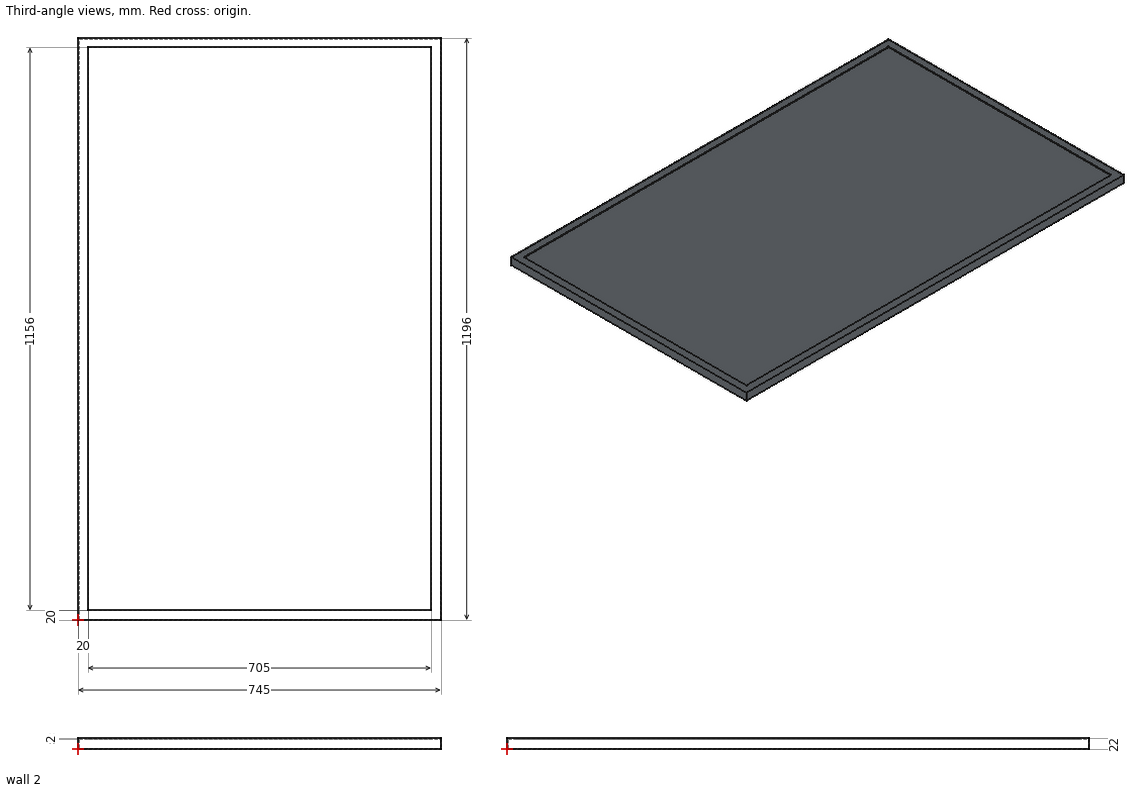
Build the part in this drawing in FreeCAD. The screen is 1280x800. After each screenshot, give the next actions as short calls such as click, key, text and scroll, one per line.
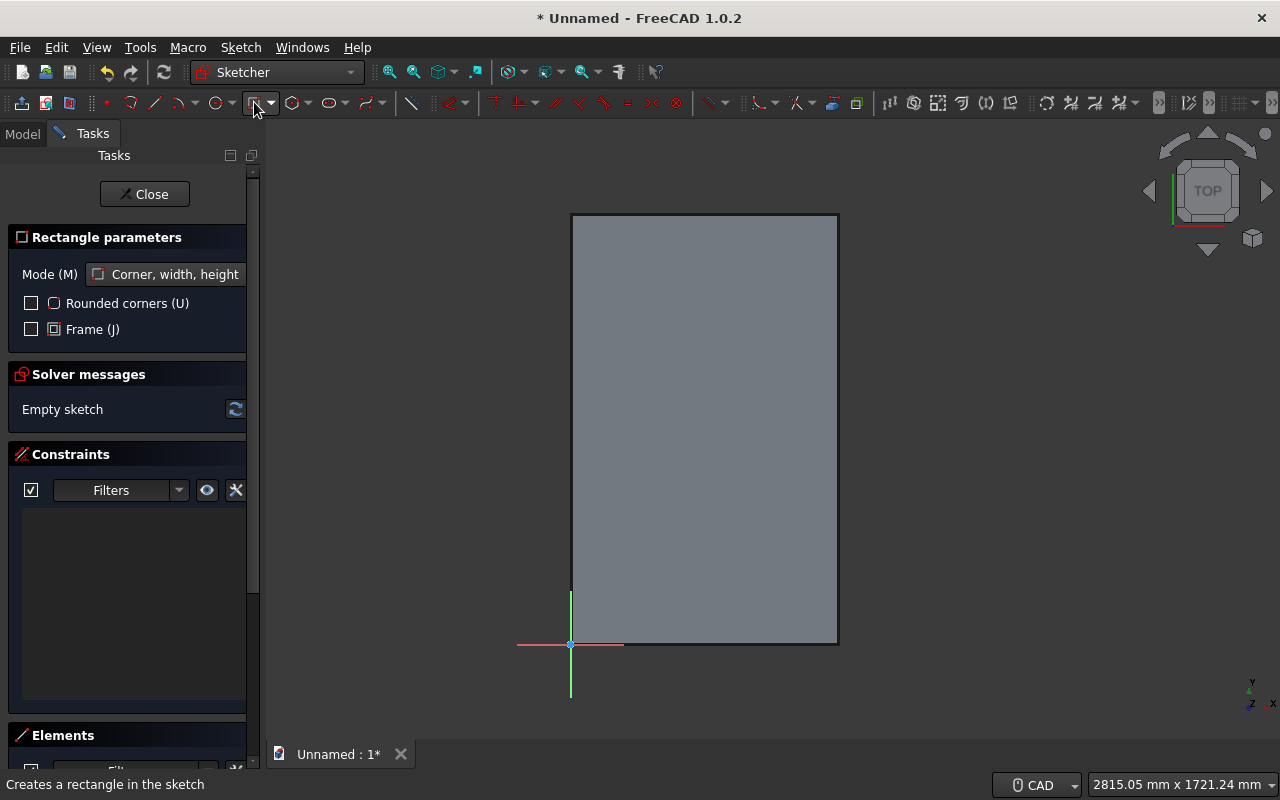
click(571, 645)
move(839, 214)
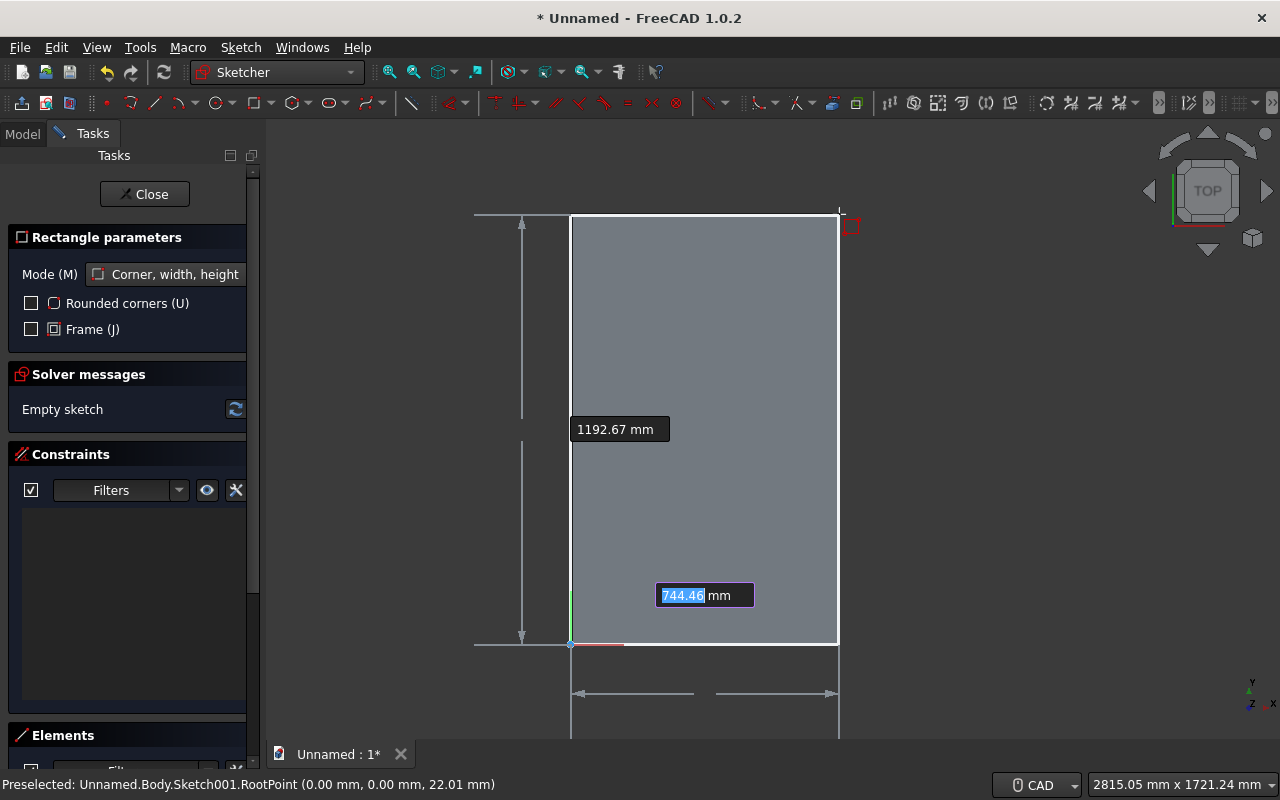
text(745)
key(Tab)
text(1196)
key(Return)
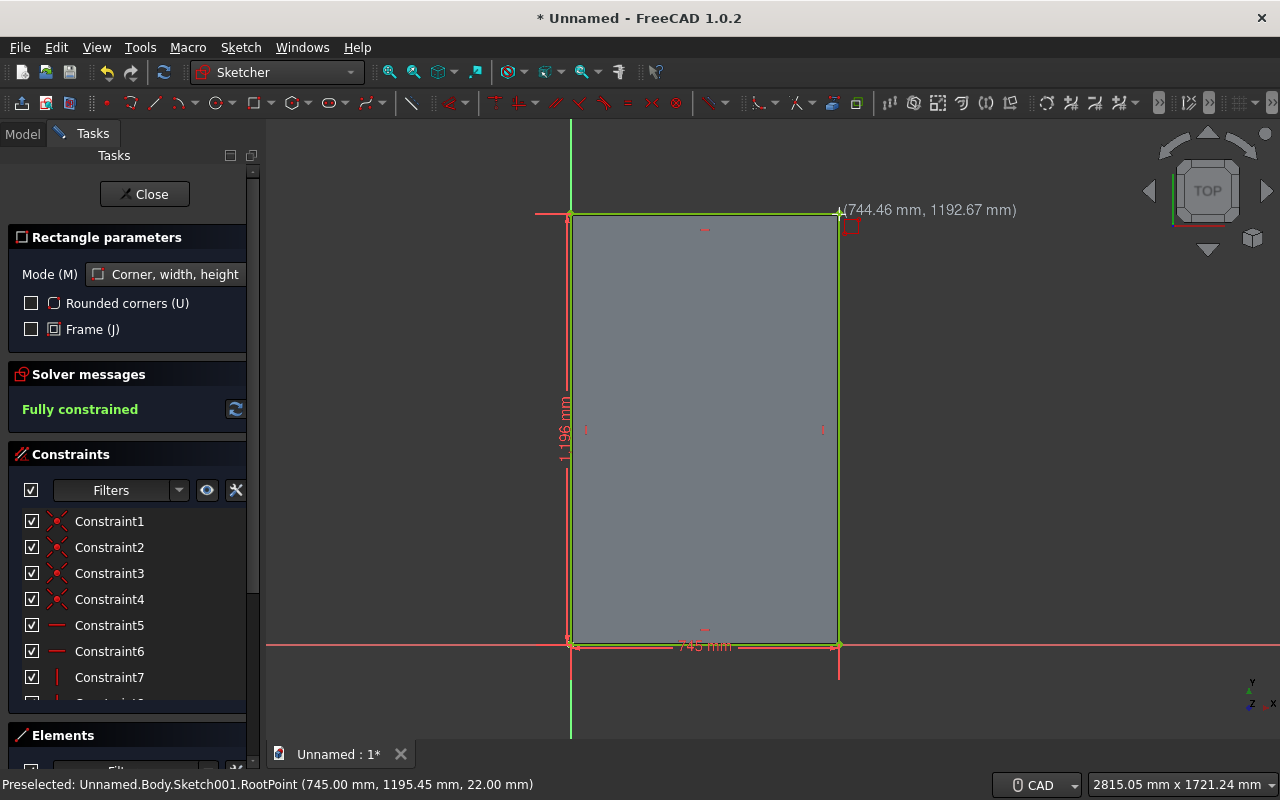
scroll(578, 221, up, 4)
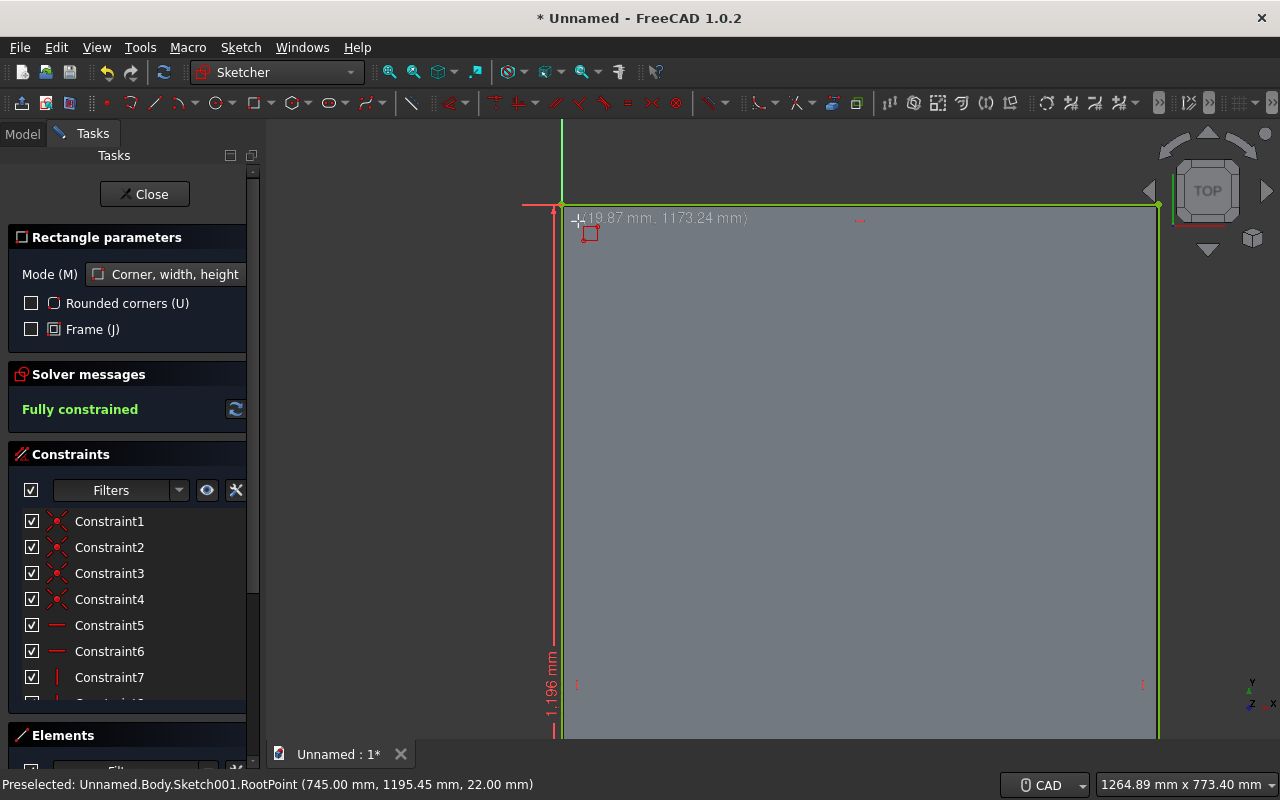
click(578, 221)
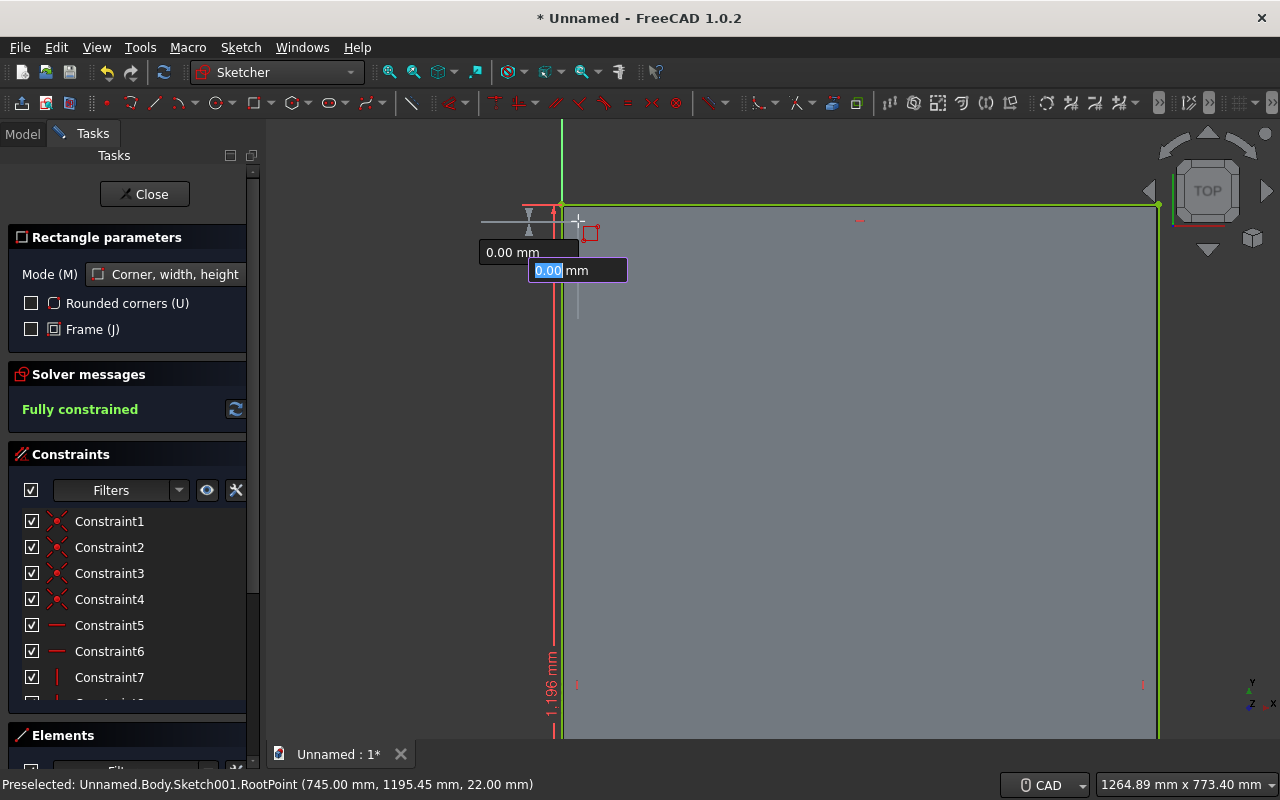
scroll(577, 221, down, 4)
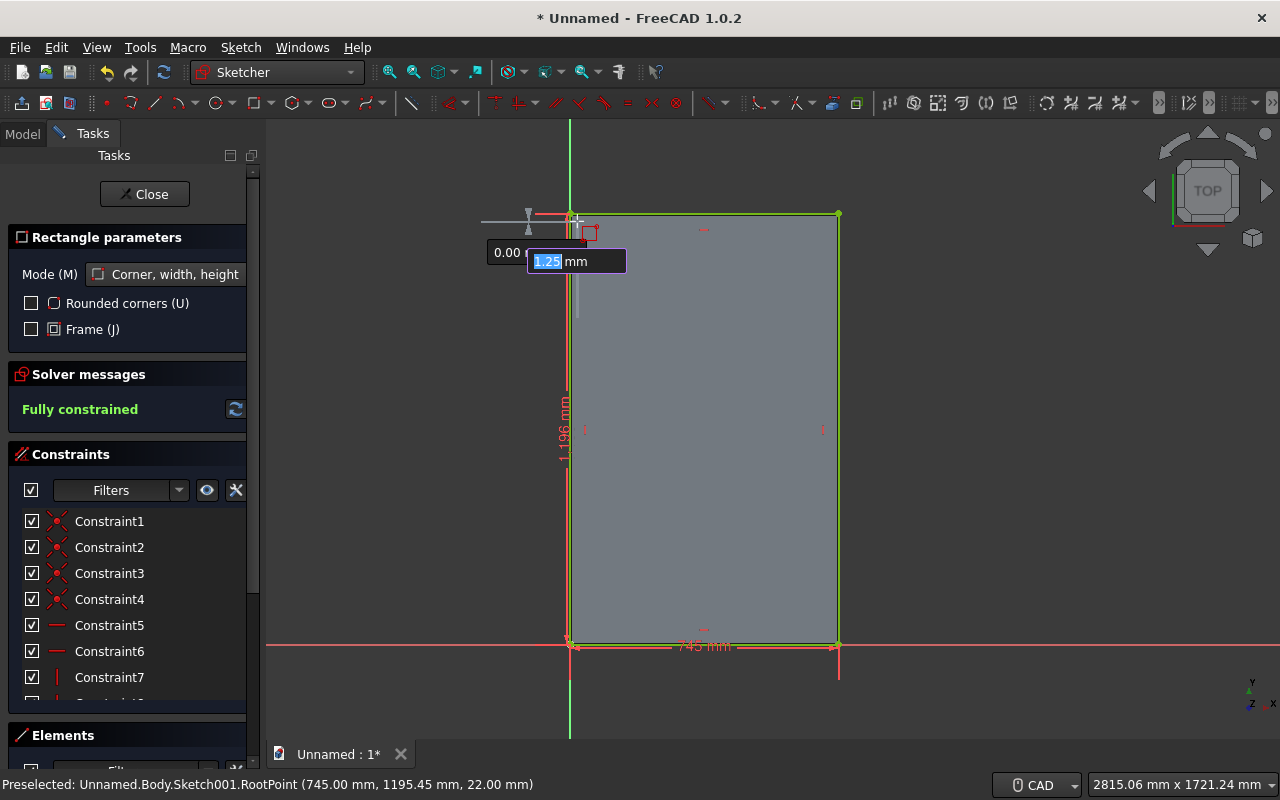
scroll(831, 637, up, 4)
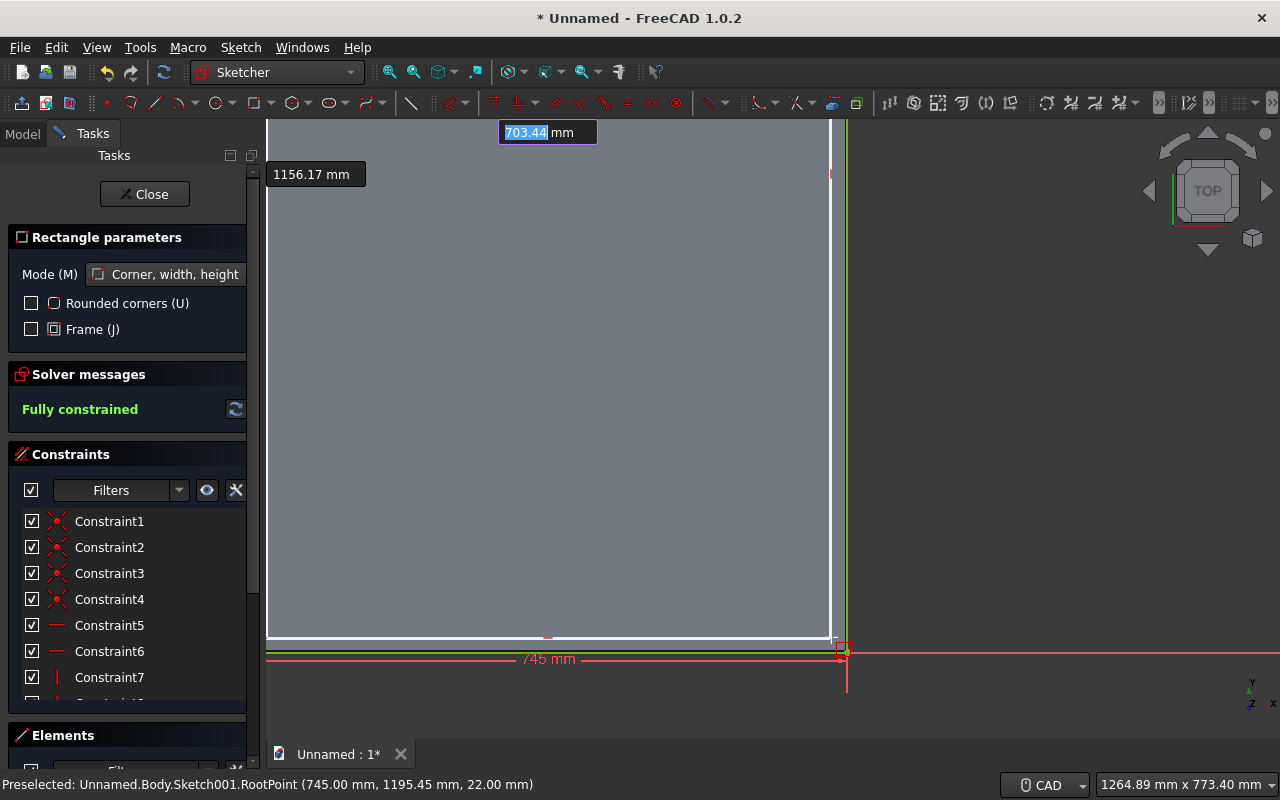
click(831, 637)
key(Escape)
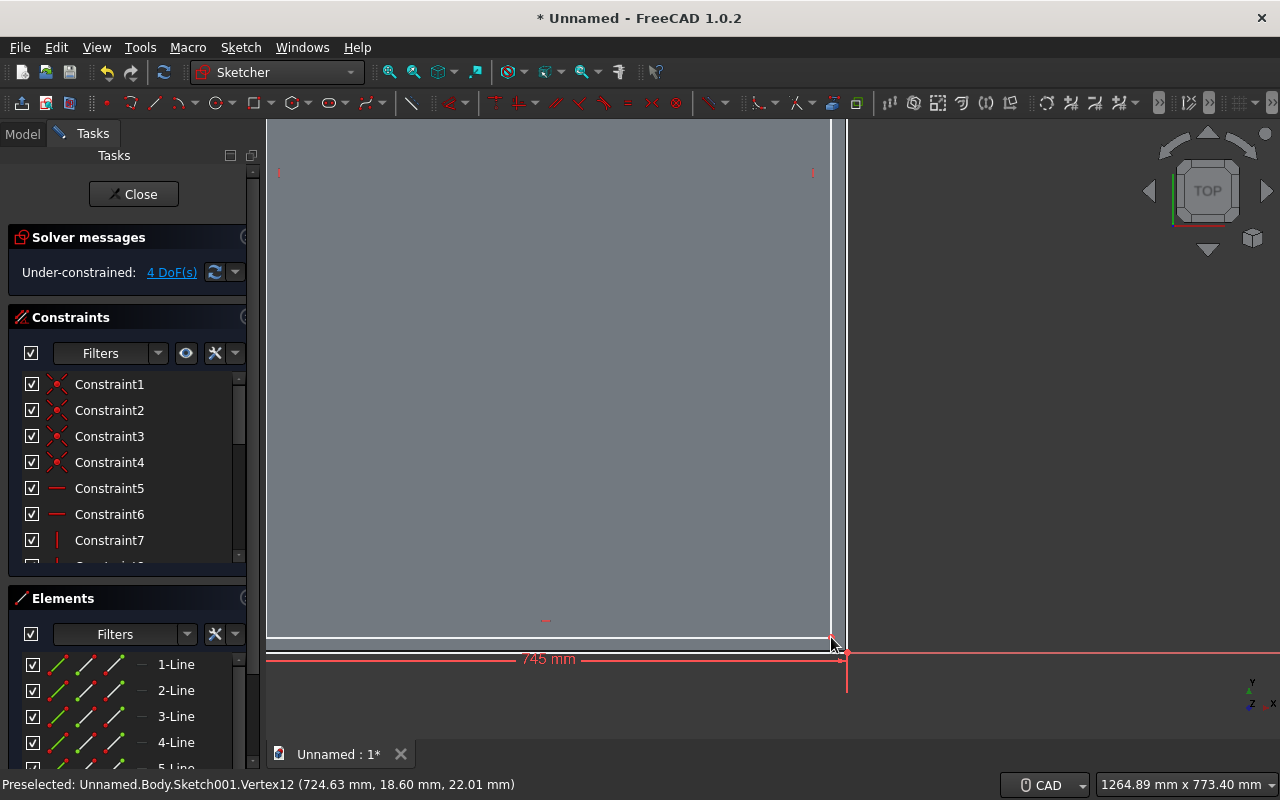
click(450, 104)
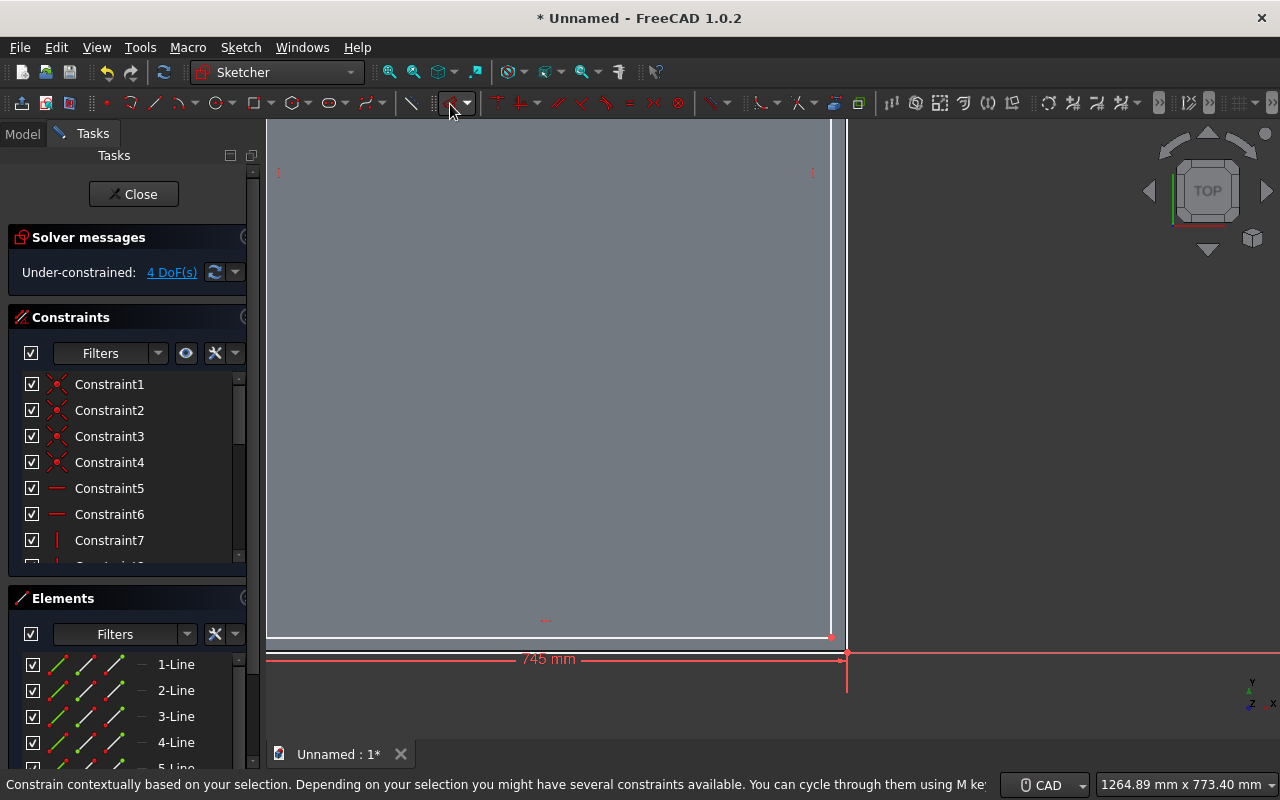
click(436, 638)
click(563, 672)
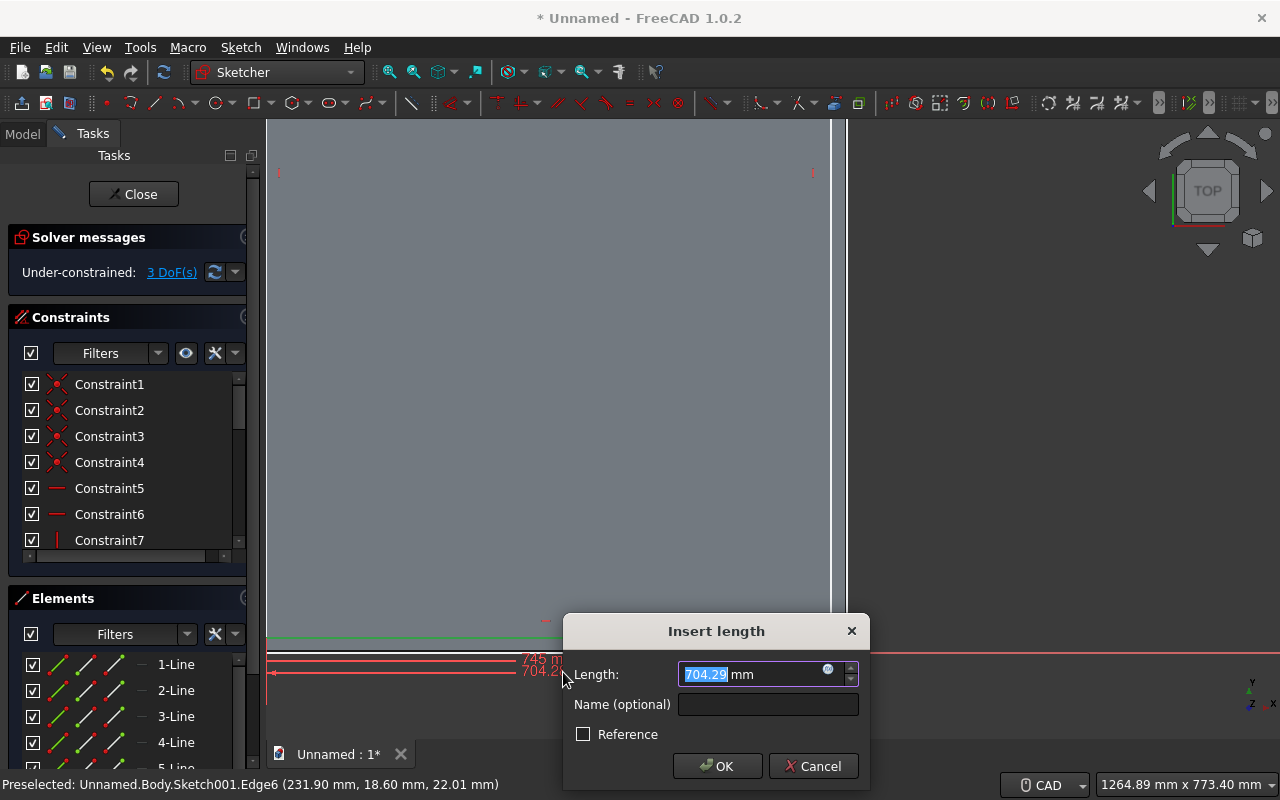
text(705)
key(Return)